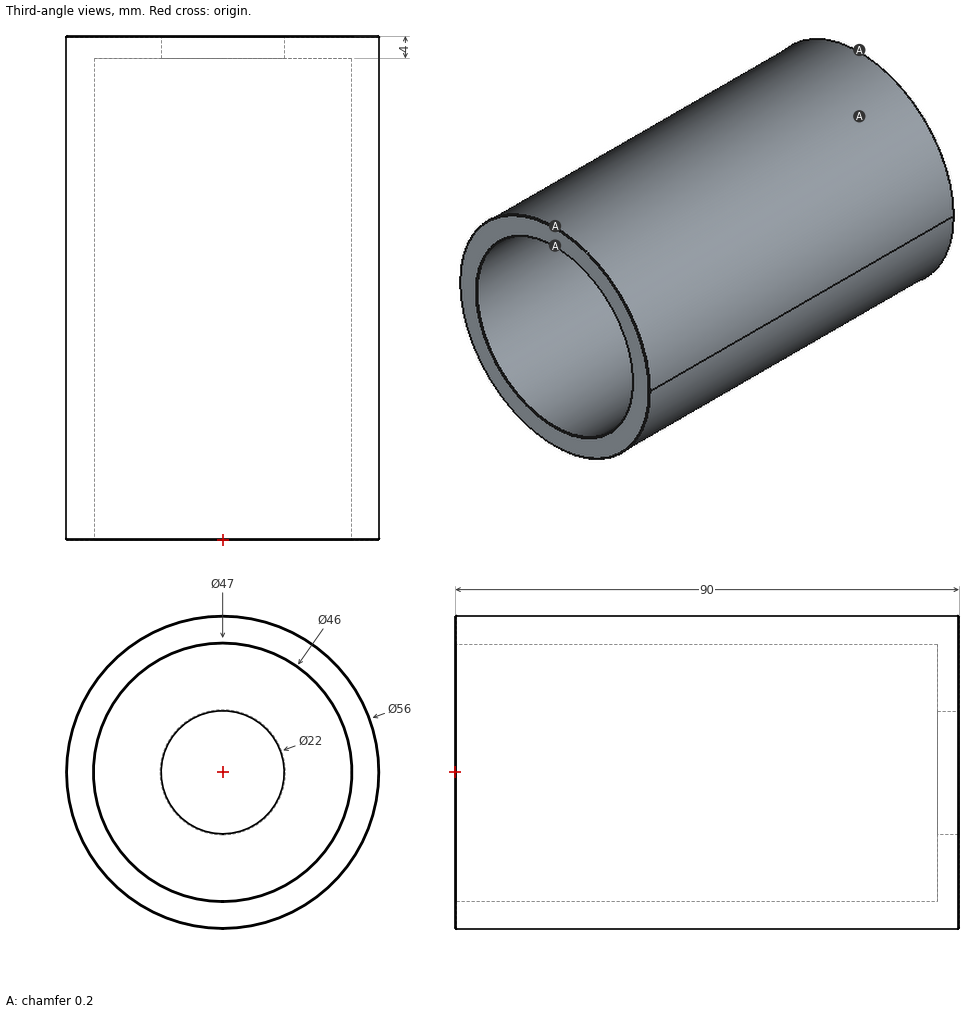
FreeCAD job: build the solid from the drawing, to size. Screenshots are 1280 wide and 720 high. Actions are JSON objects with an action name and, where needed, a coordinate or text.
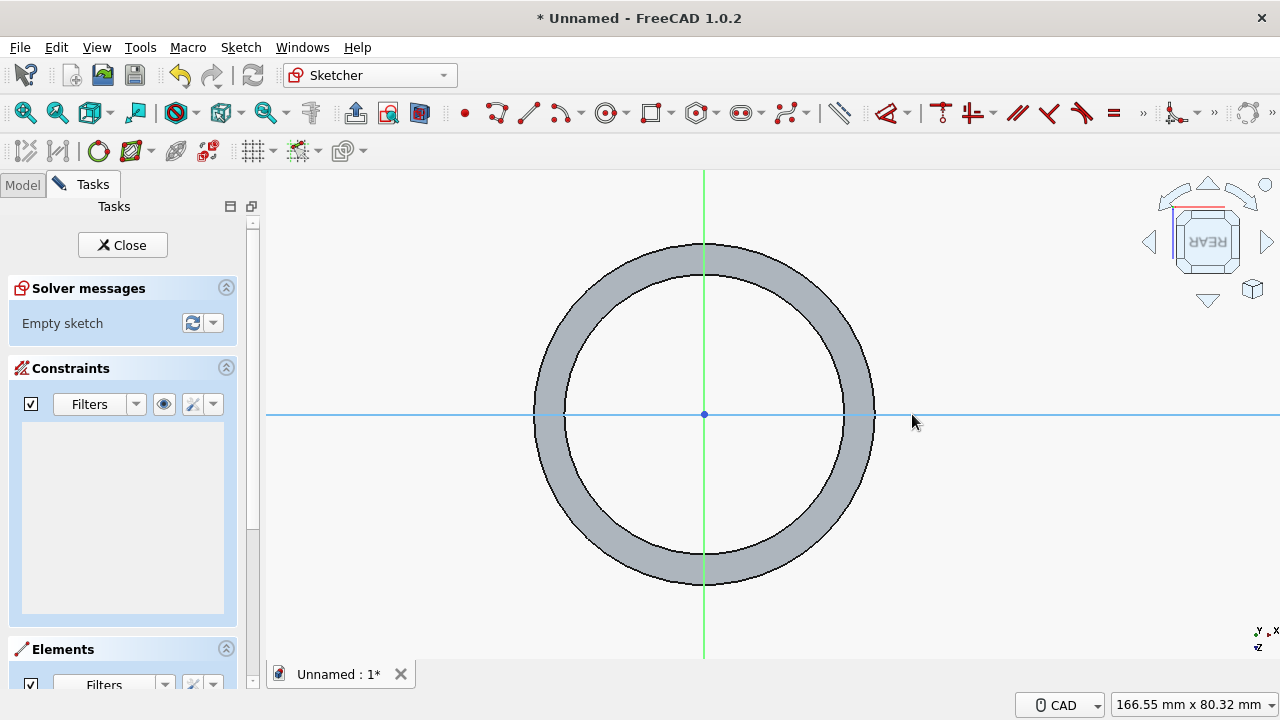
{"action": "key", "text": "g c"}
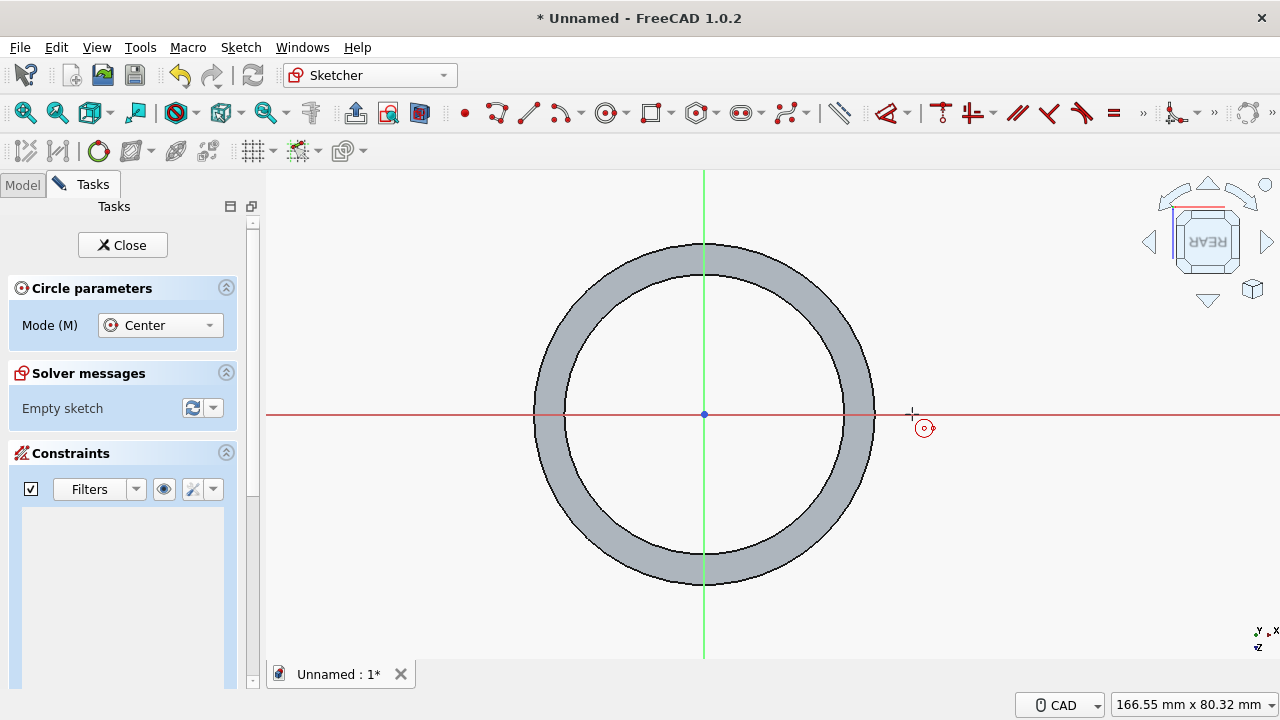
{"action": "left_click", "coordinate": [704, 414]}
{"action": "left_click", "coordinate": [805, 313]}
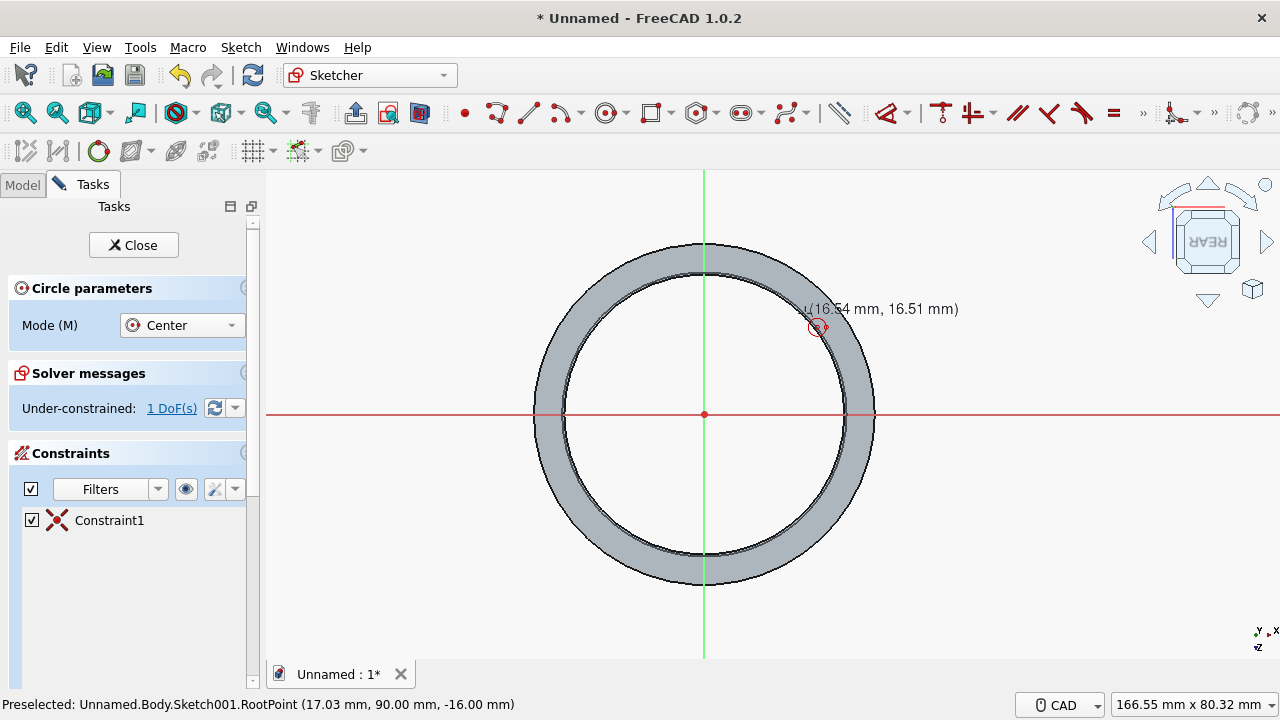
{"action": "left_click", "coordinate": [704, 414]}
{"action": "left_click", "coordinate": [752, 367]}
{"action": "key", "text": "Escape"}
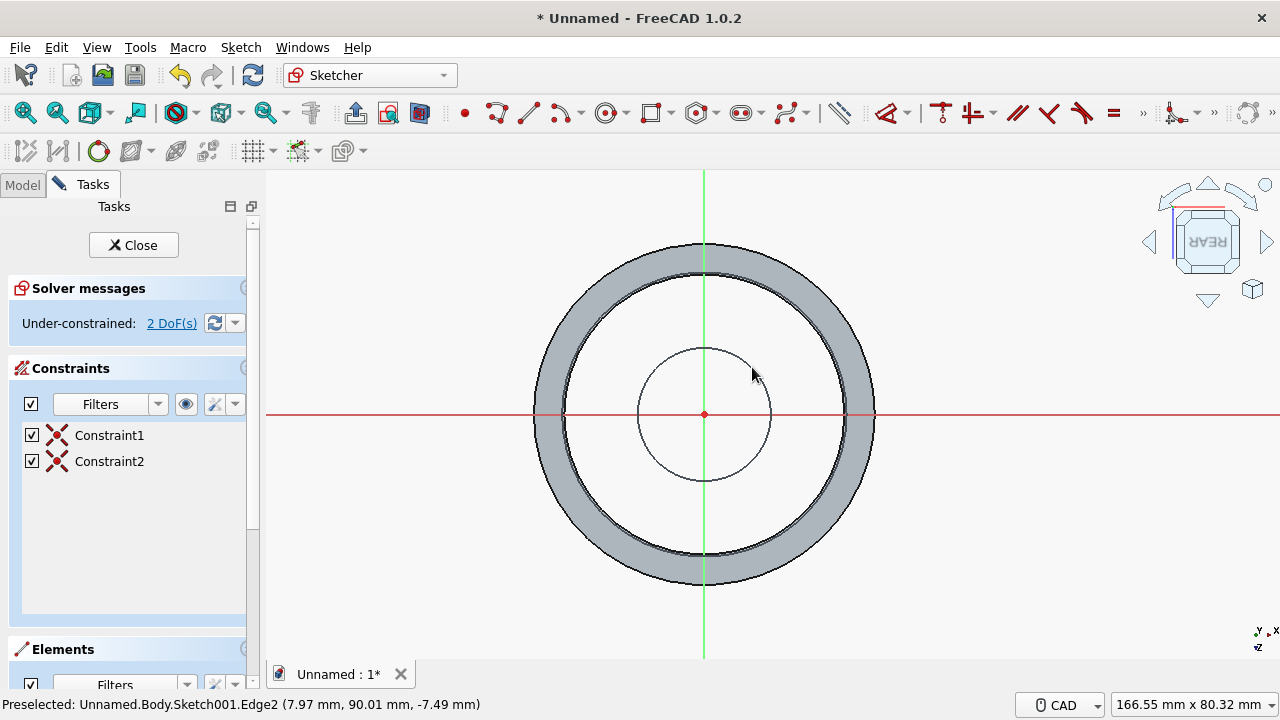
{"action": "key", "text": "d"}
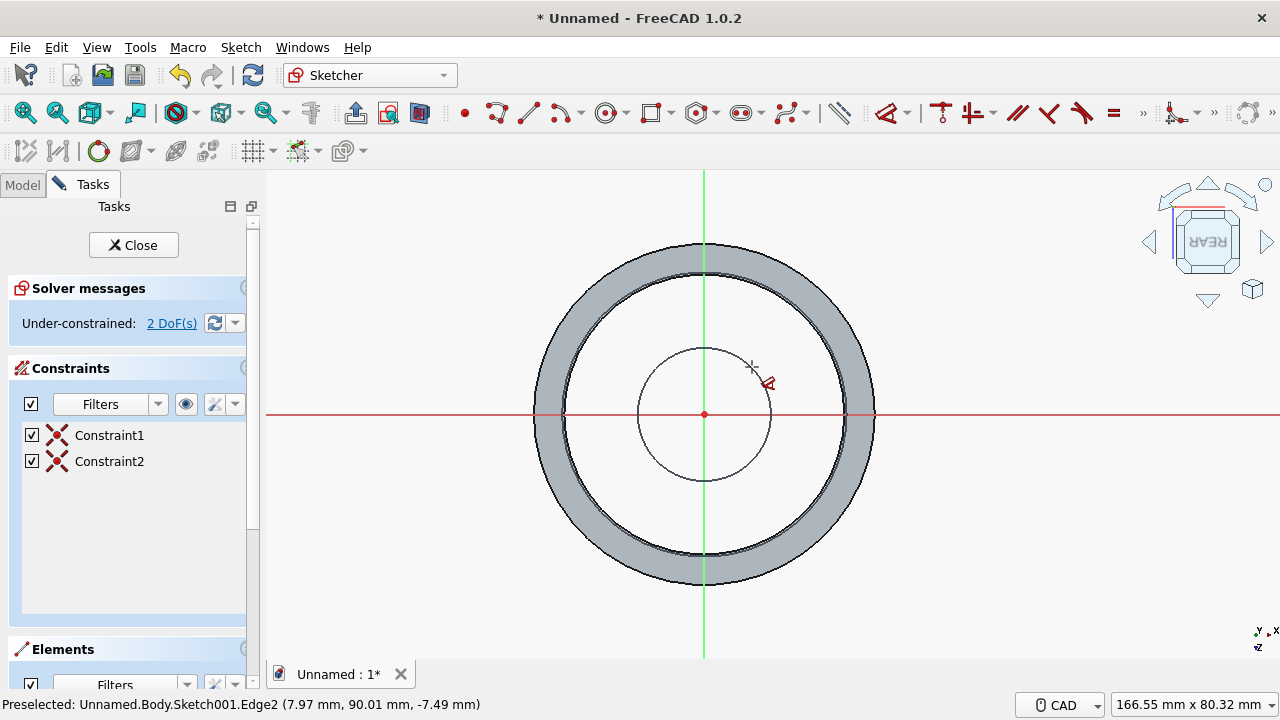
{"action": "left_click", "coordinate": [805, 314]}
{"action": "left_click", "coordinate": [828, 291]}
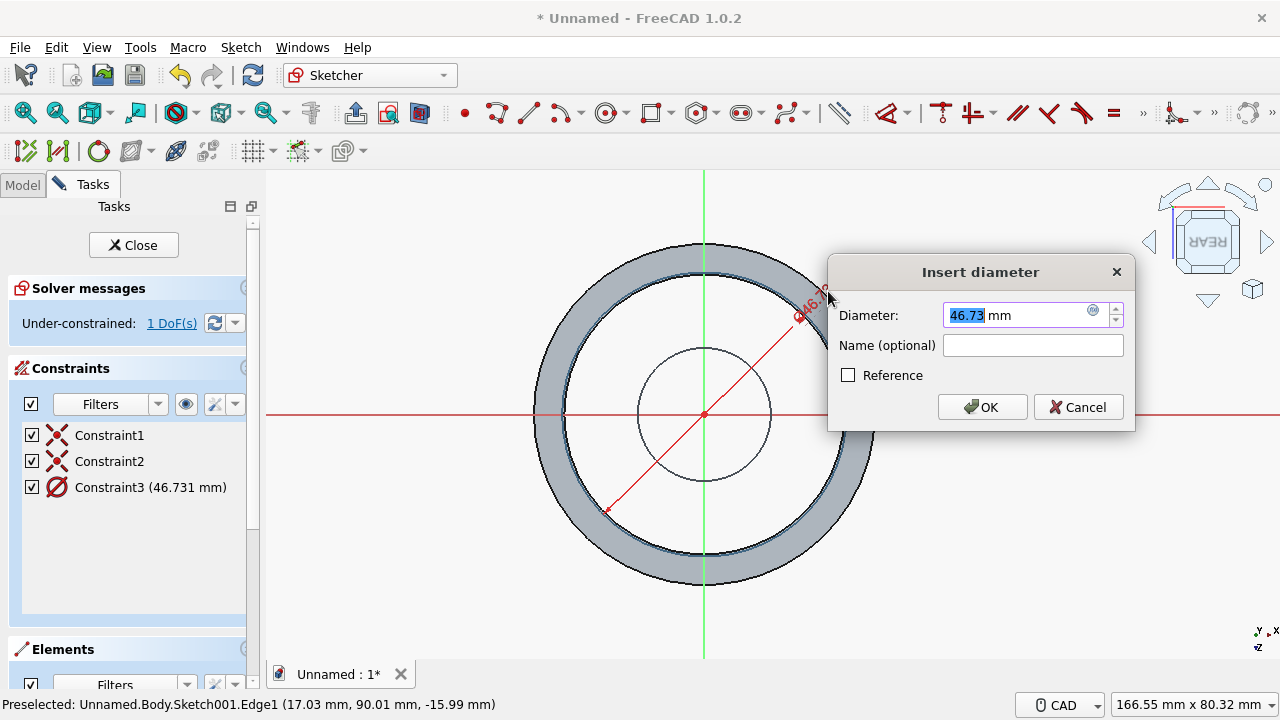
{"action": "type", "text": "47"}
{"action": "key", "text": "Return"}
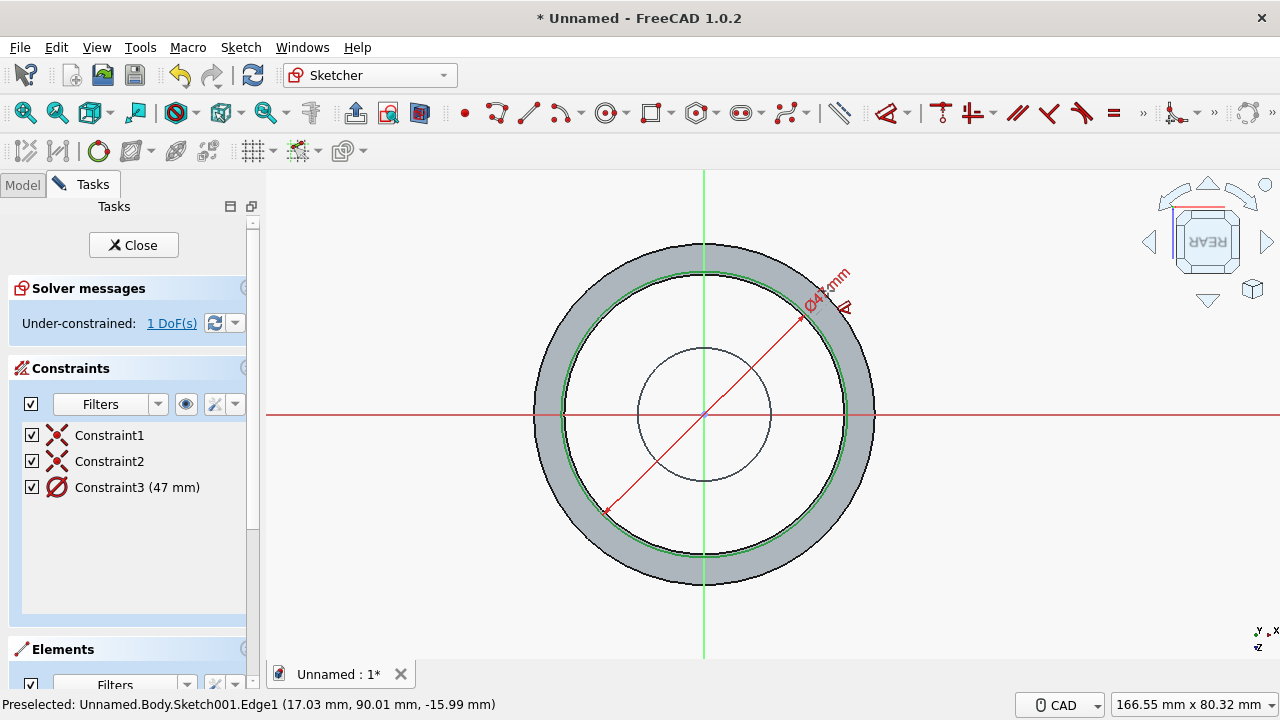
{"action": "left_click", "coordinate": [751, 367]}
{"action": "left_click", "coordinate": [773, 344]}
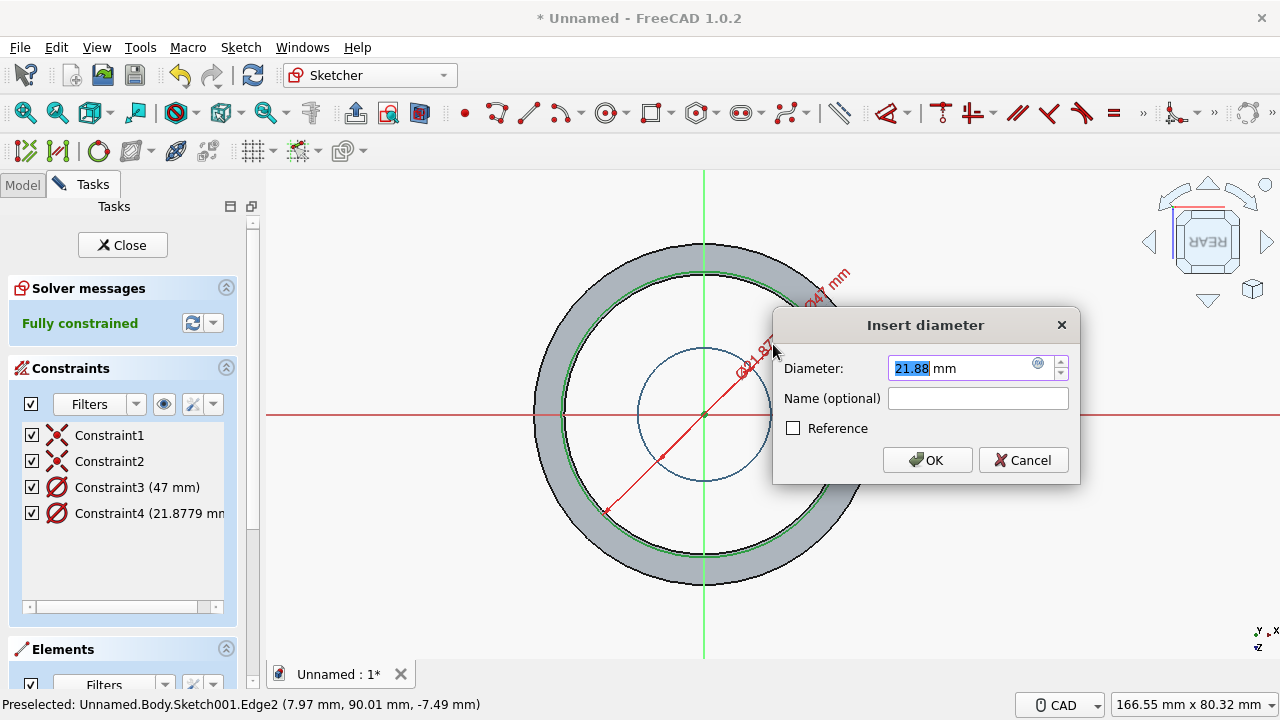
{"action": "type", "text": "22"}
{"action": "key", "text": "Return"}
{"action": "key", "text": "Escape"}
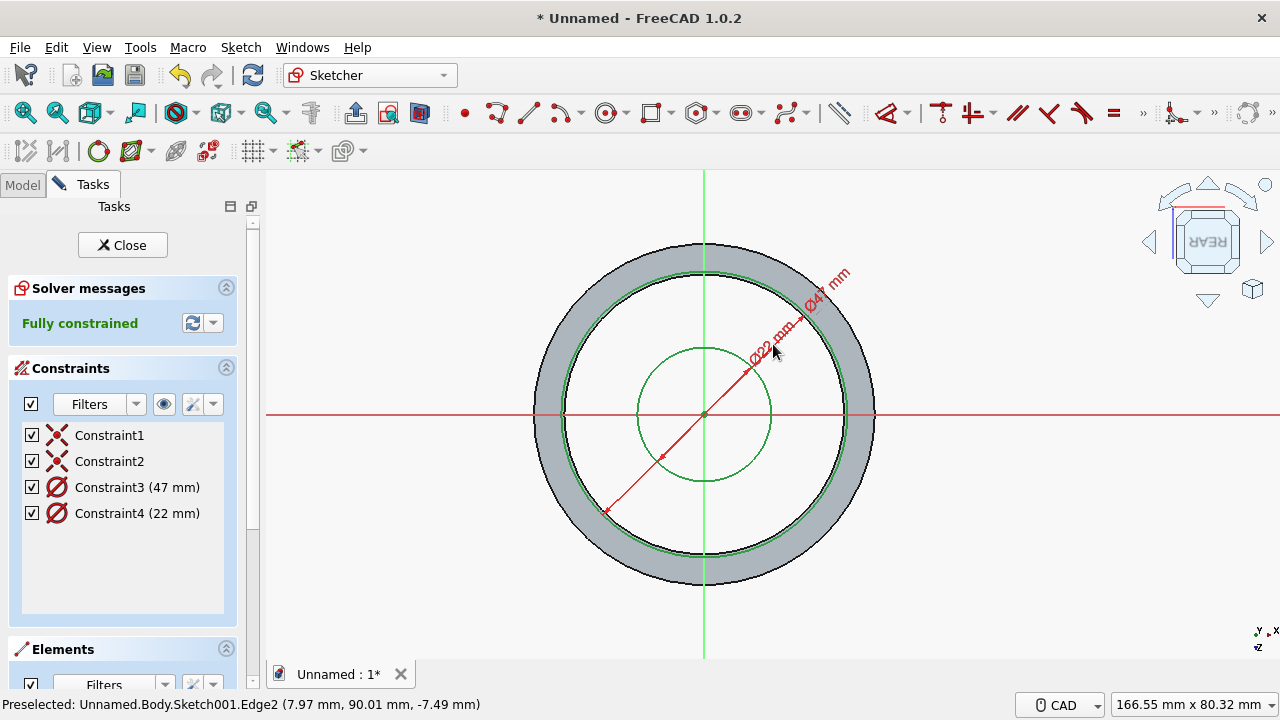
{"action": "left_click", "coordinate": [123, 245]}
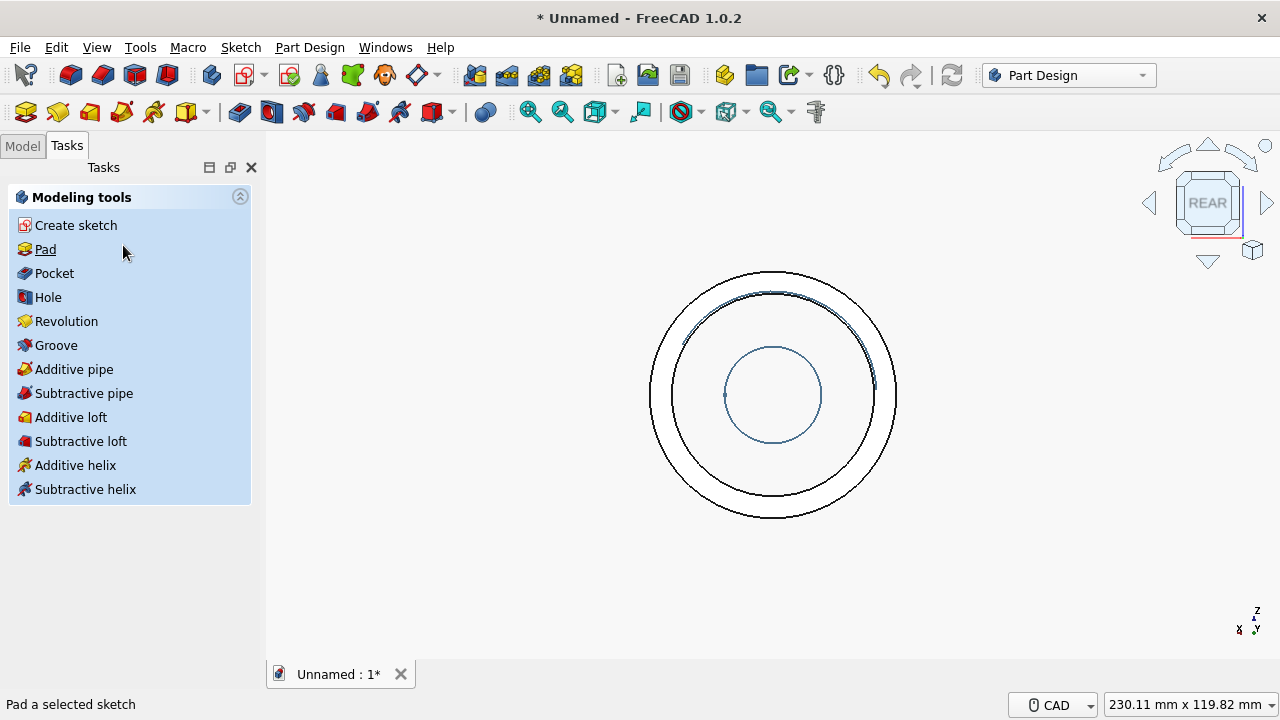
{"action": "left_click", "coordinate": [26, 112]}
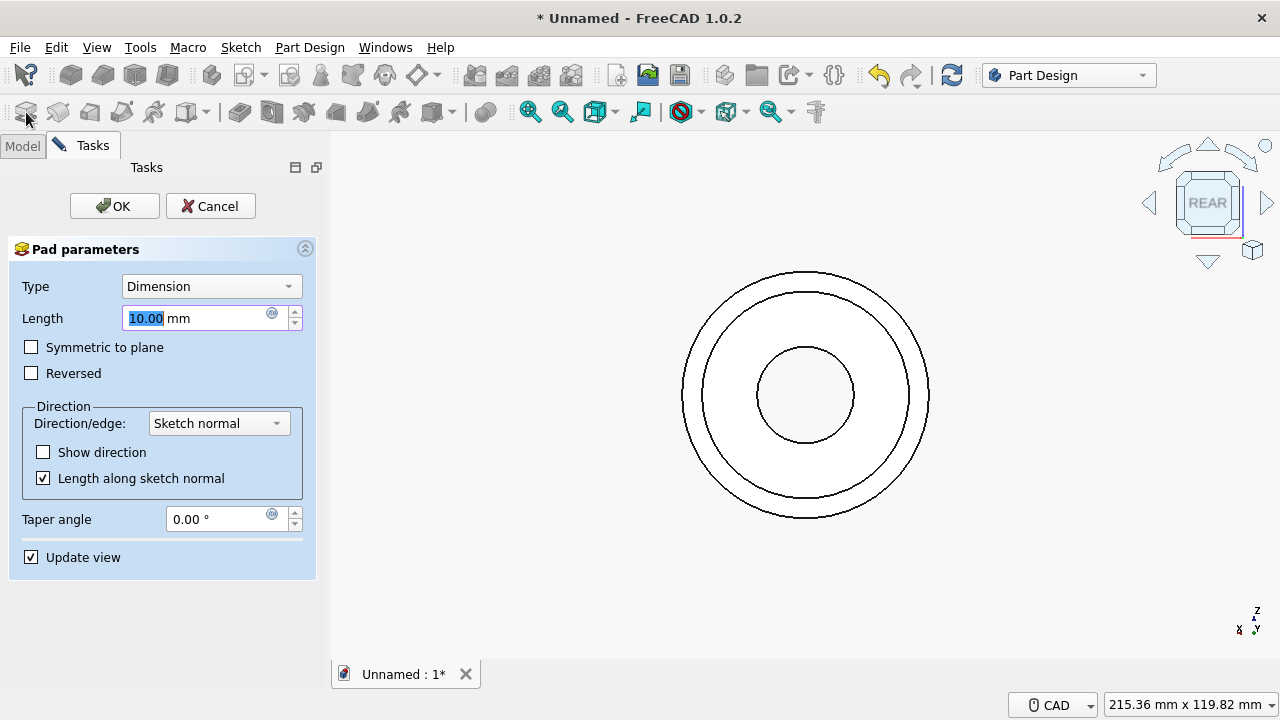
{"action": "type", "text": "4"}
{"action": "key", "text": "Tab"}